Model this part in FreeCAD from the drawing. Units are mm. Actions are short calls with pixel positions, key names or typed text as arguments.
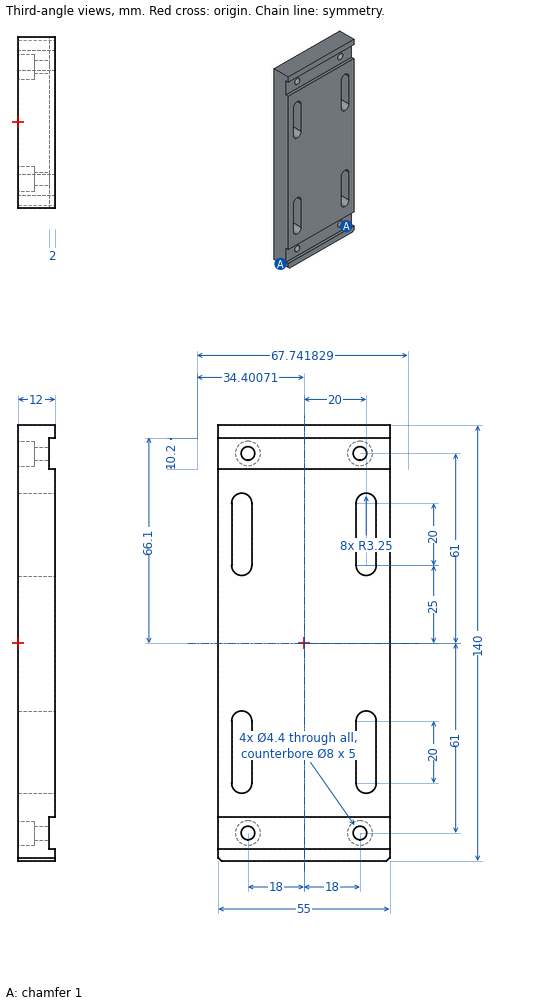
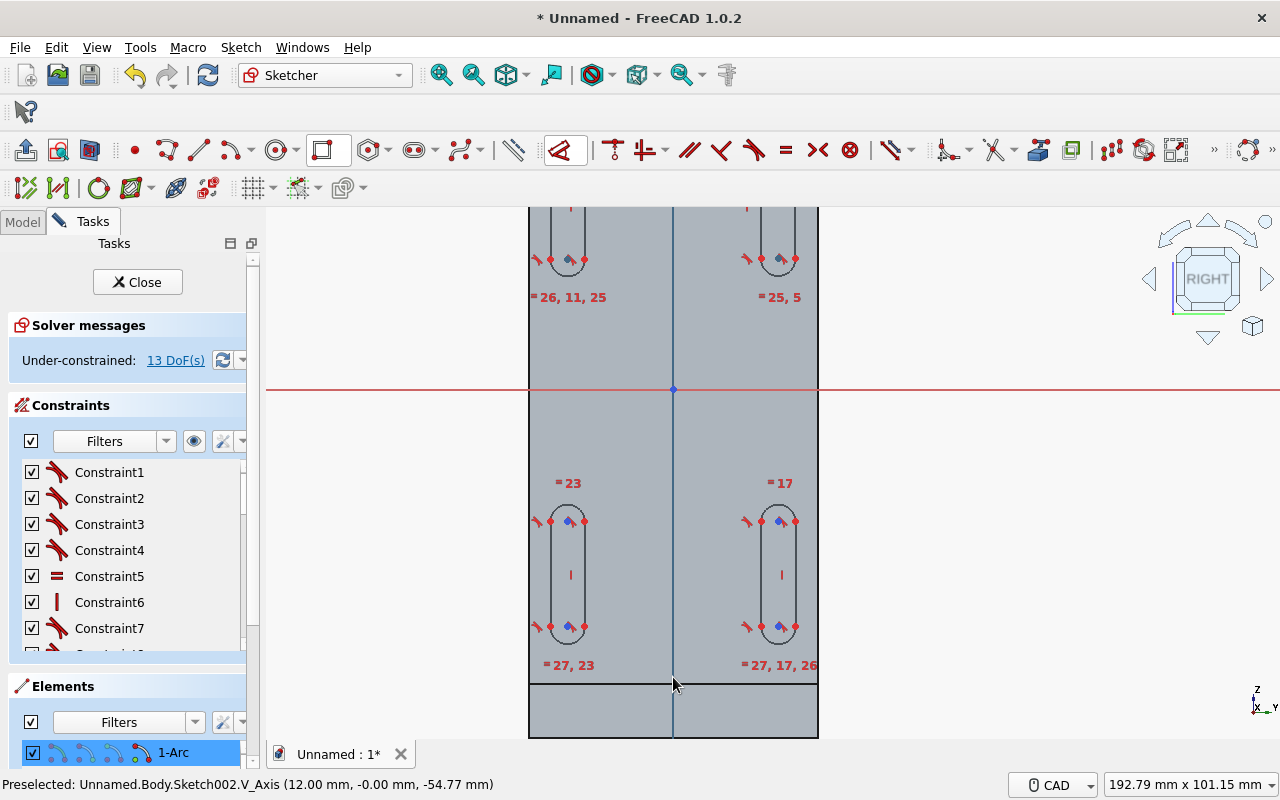
click(818, 150)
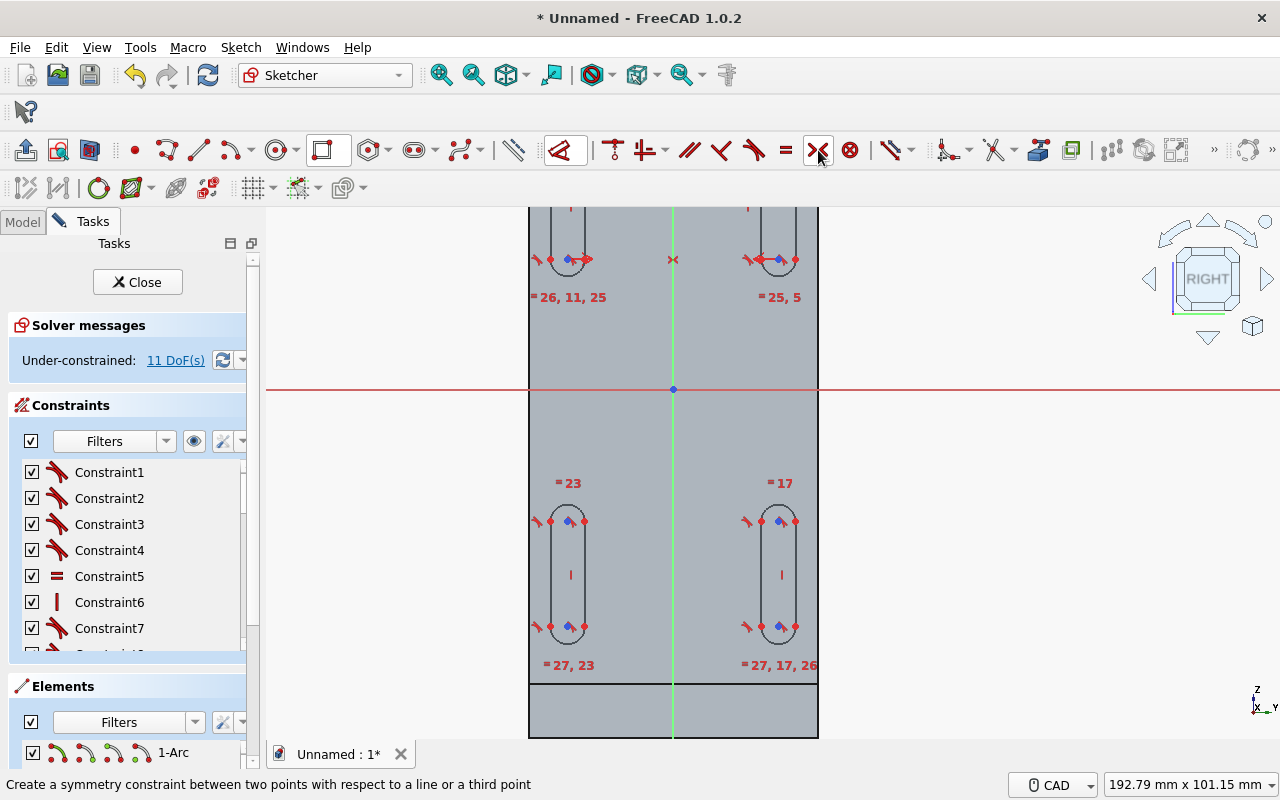
scroll(768, 642, down, 2)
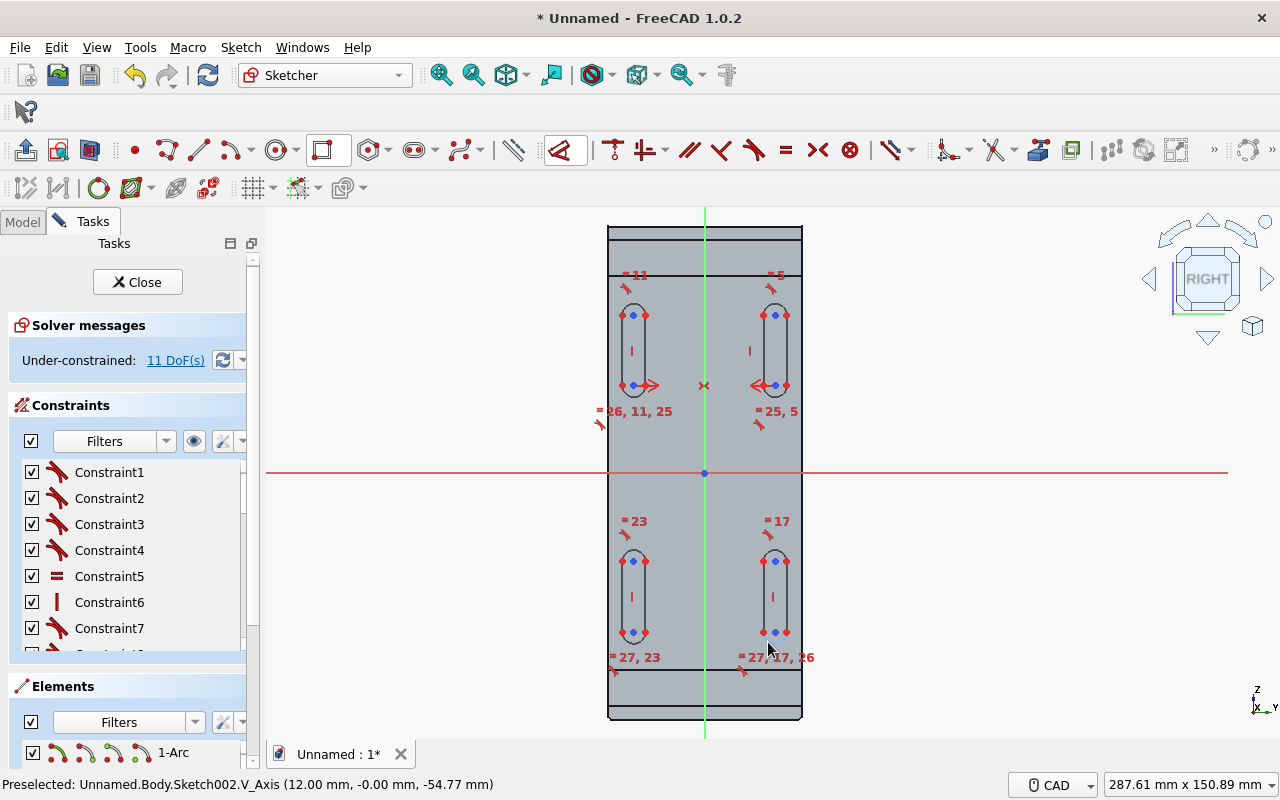
click(775, 315)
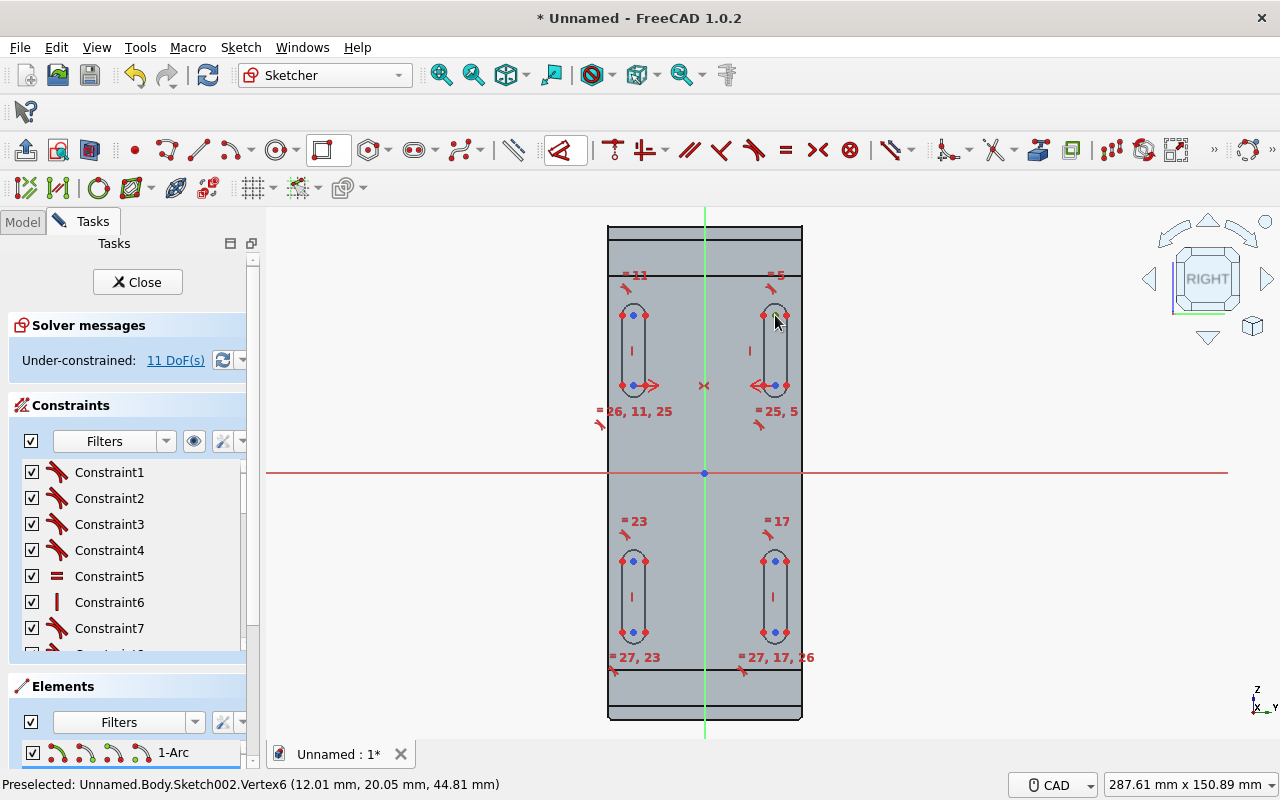
click(775, 632)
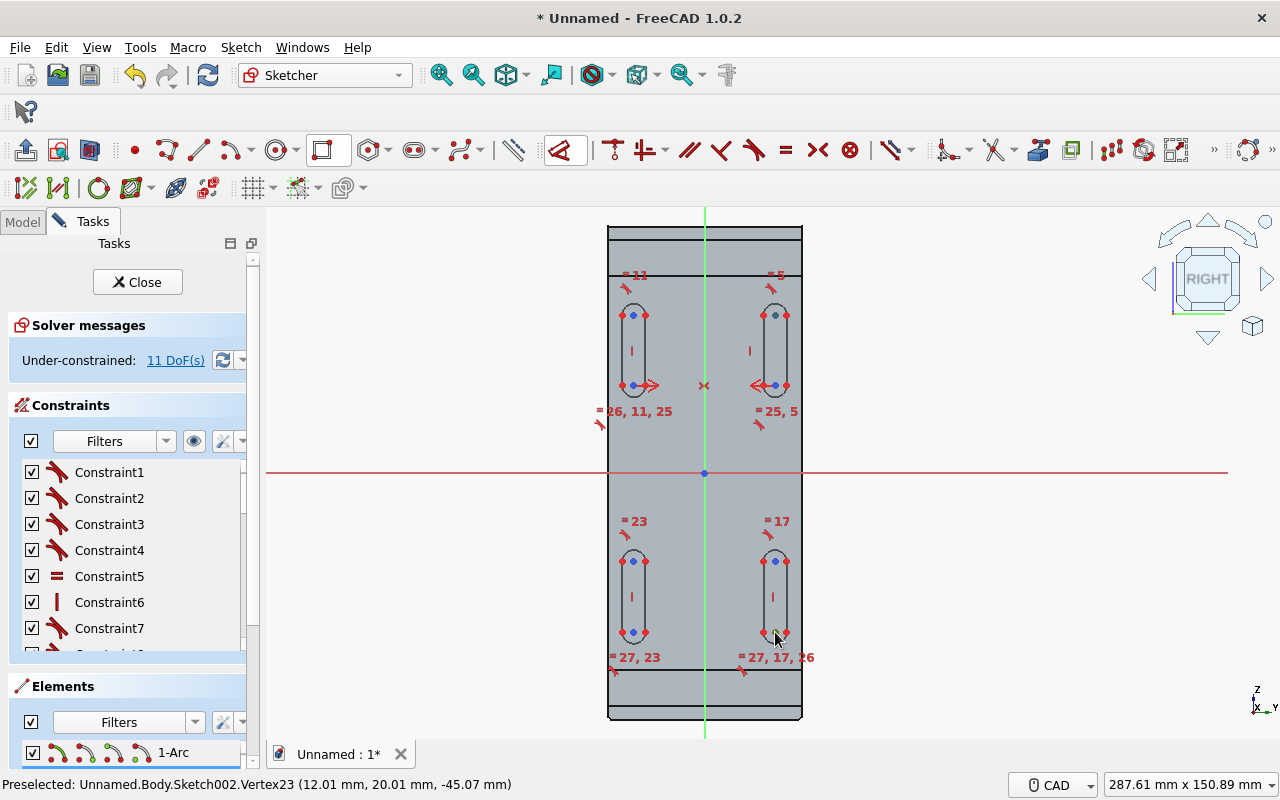
click(353, 473)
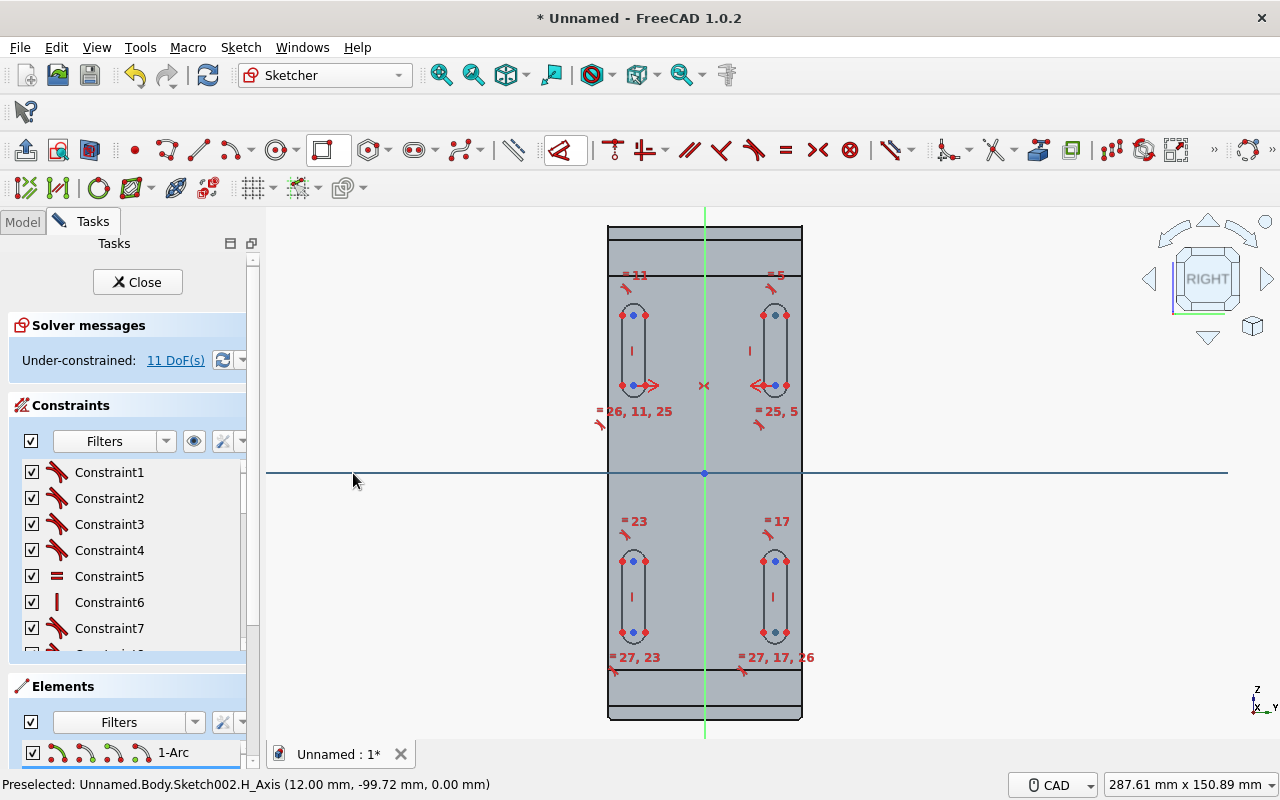
click(818, 150)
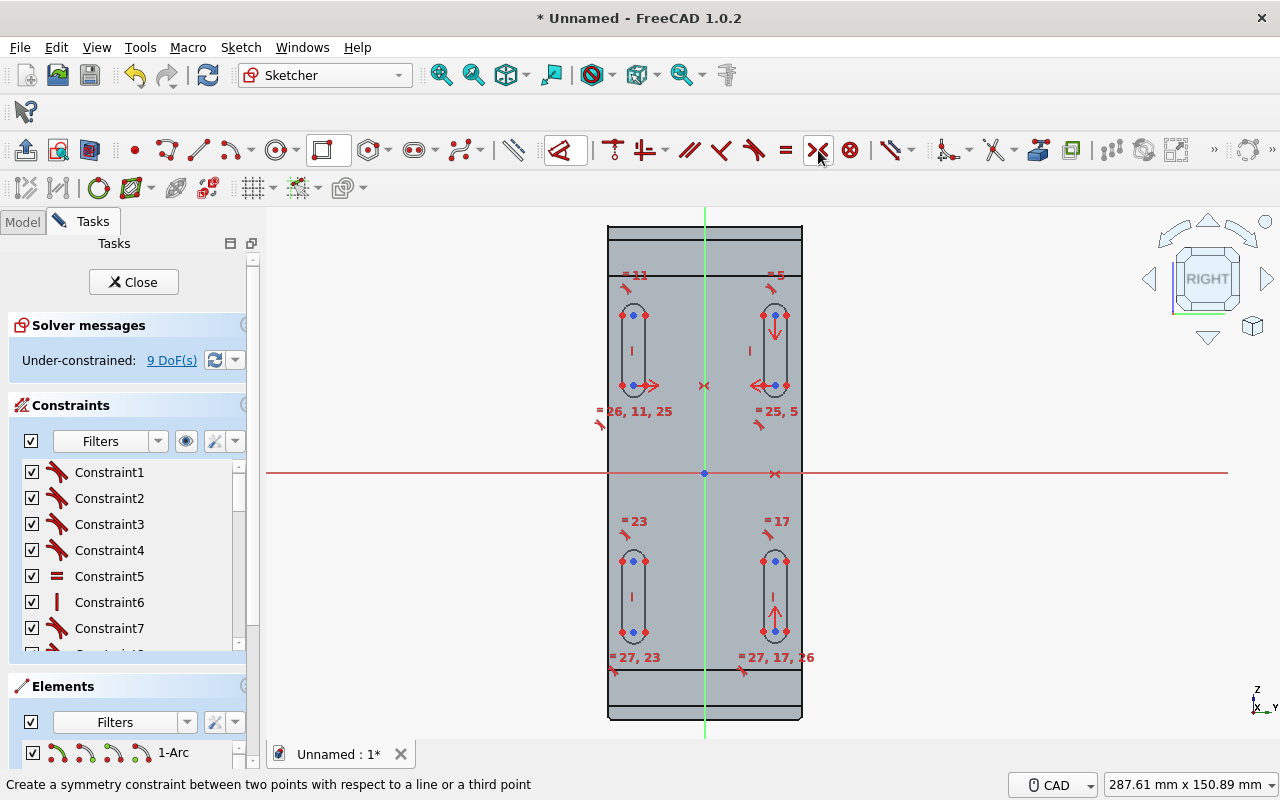
click(634, 315)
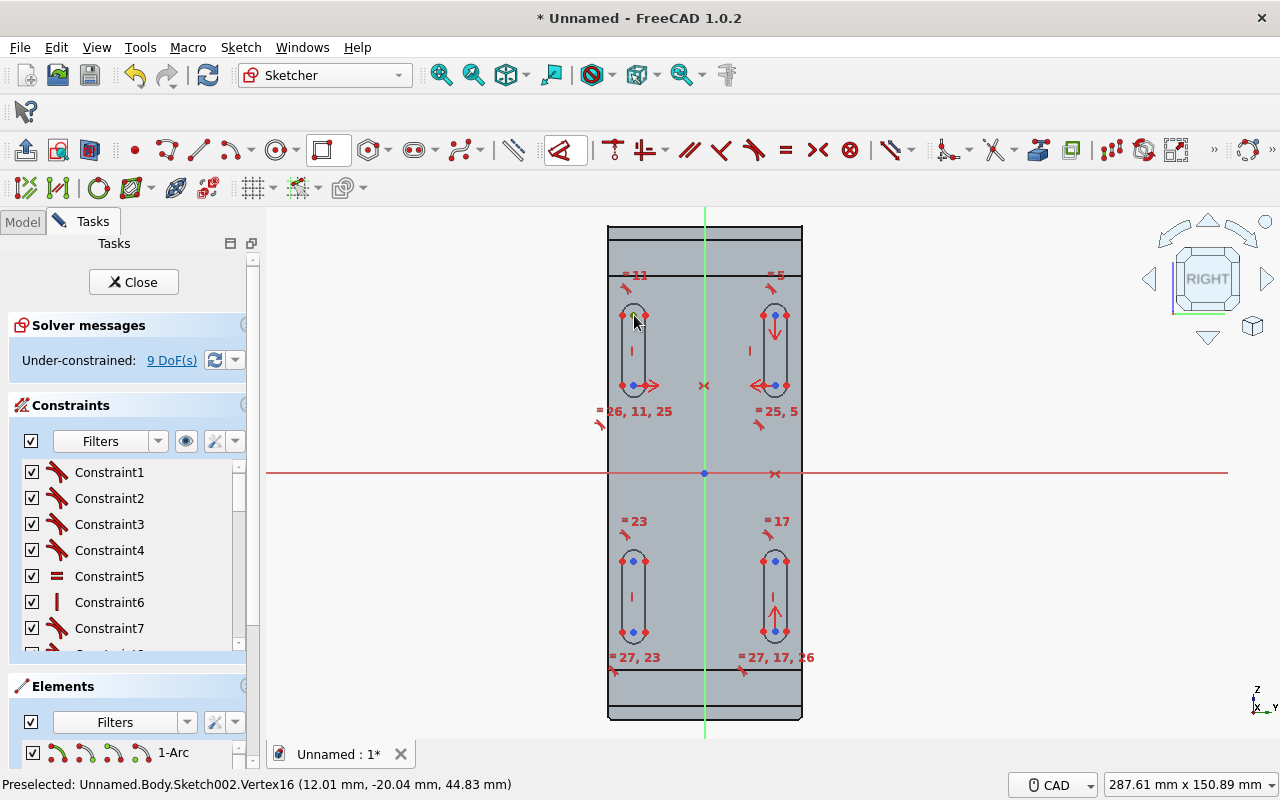
click(634, 632)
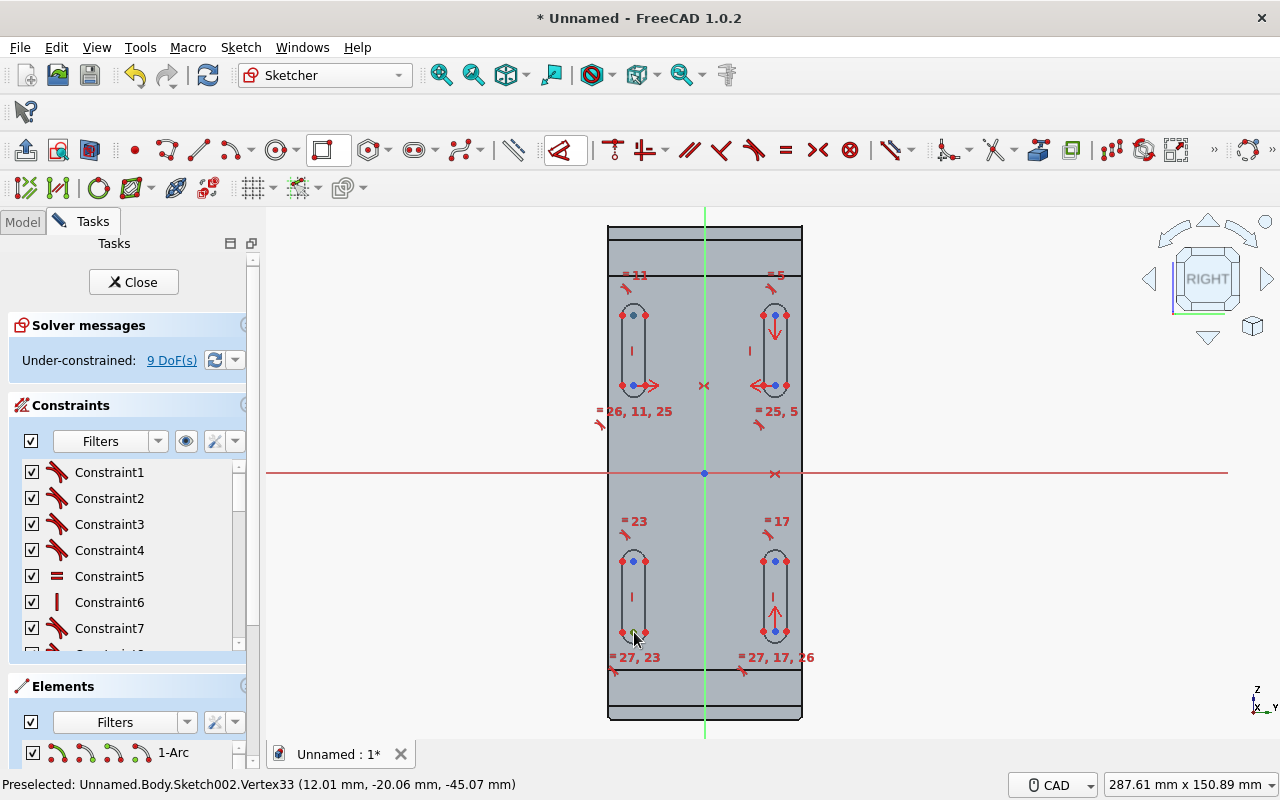
click(353, 473)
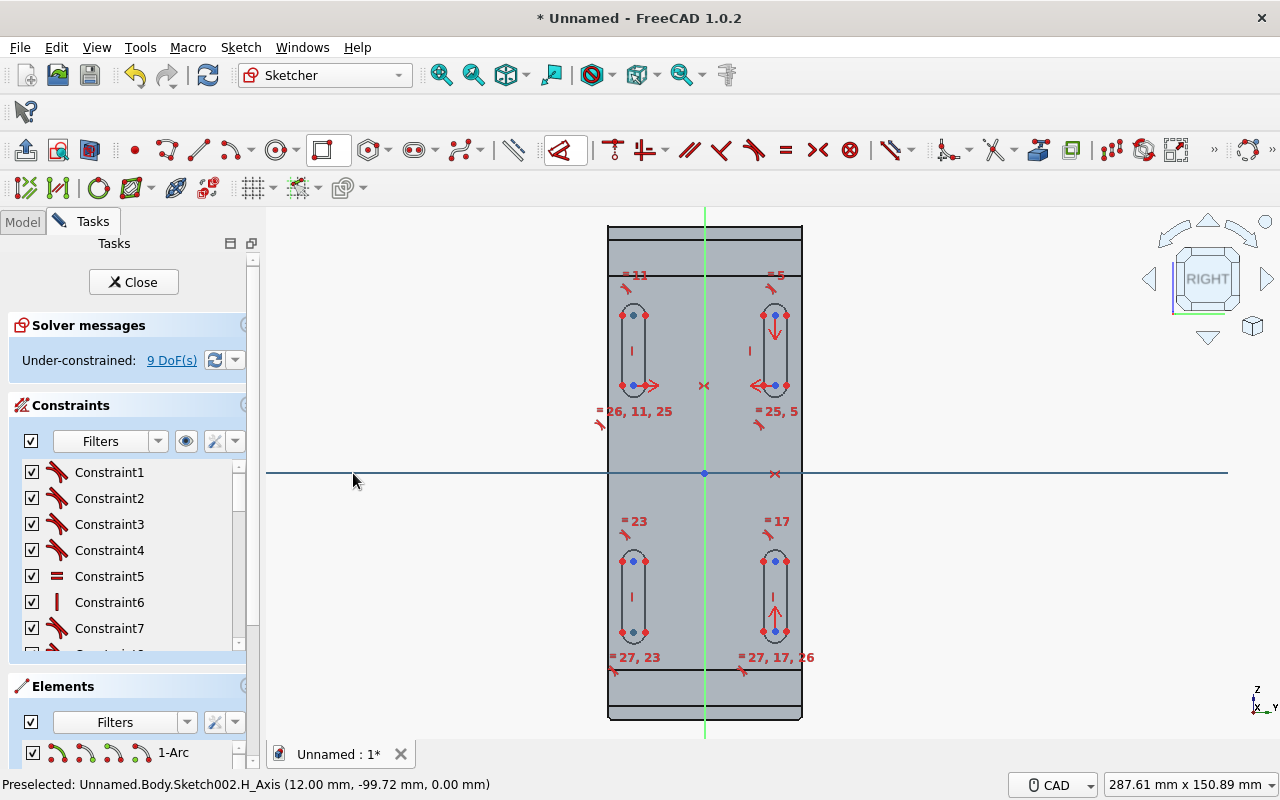
click(818, 150)